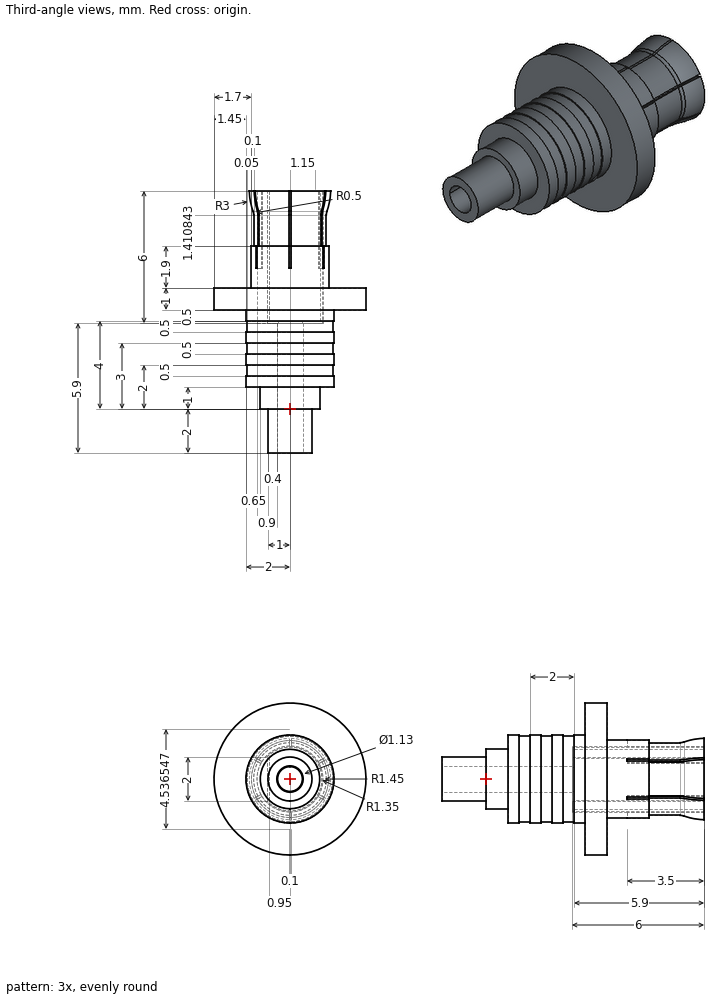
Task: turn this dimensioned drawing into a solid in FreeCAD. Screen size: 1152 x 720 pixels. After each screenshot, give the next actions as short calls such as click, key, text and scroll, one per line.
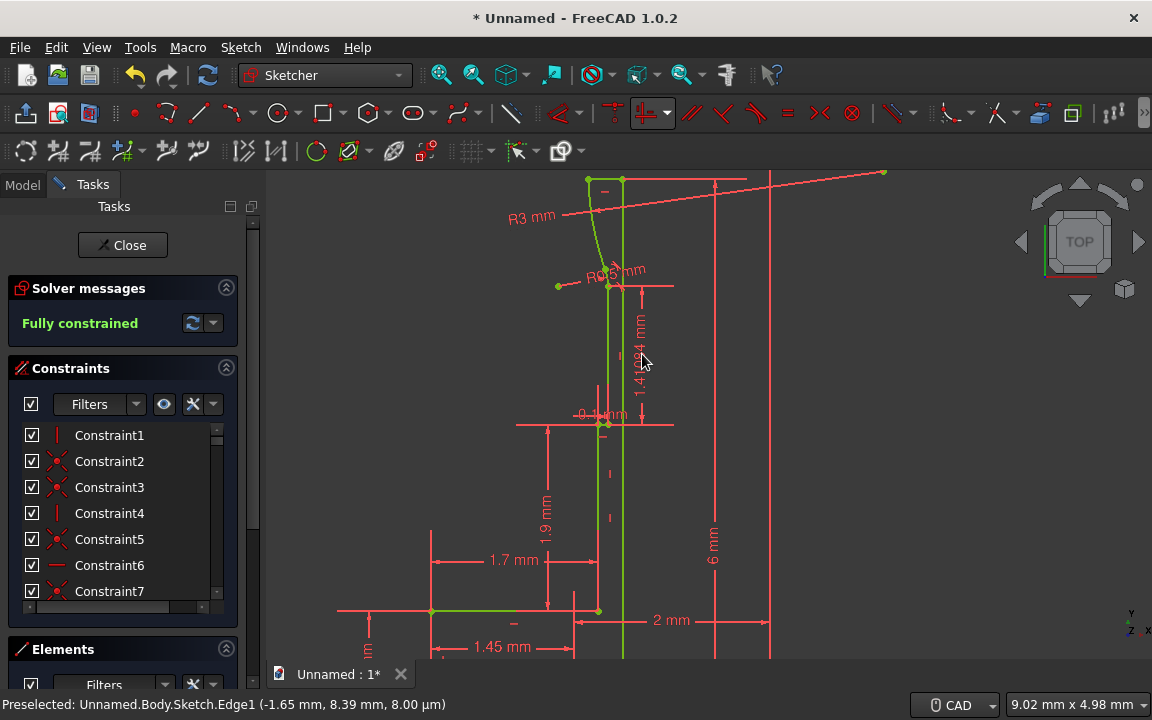
click(123, 245)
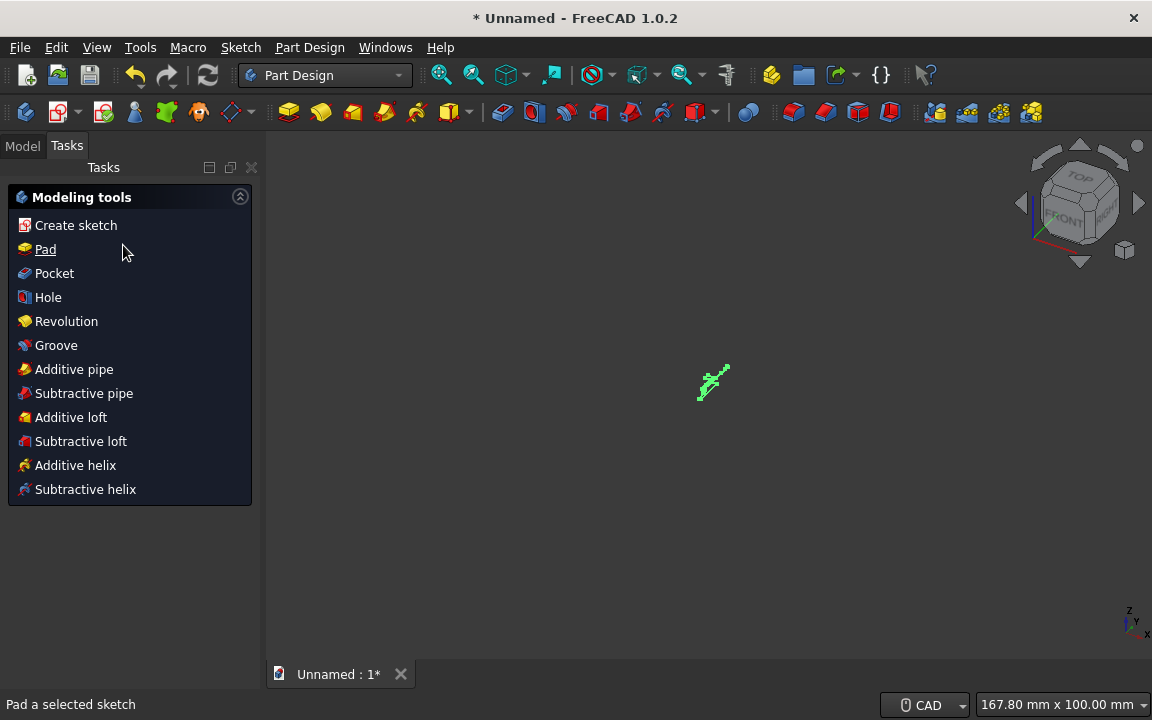
click(322, 112)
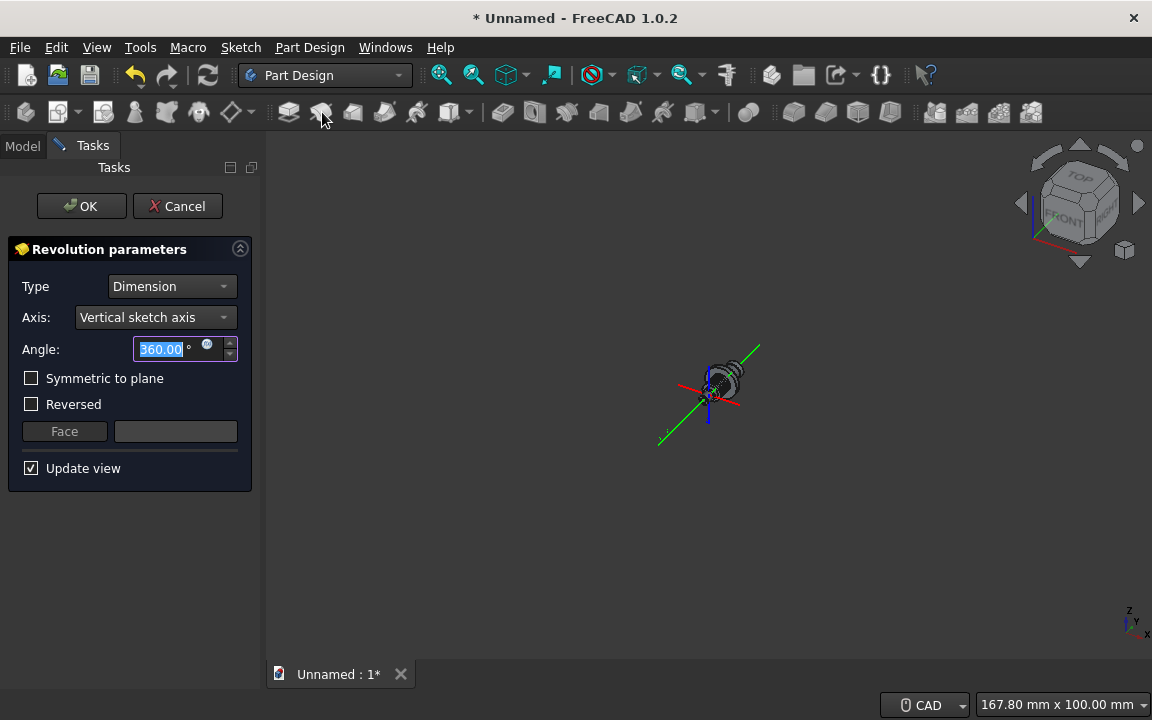
click(82, 206)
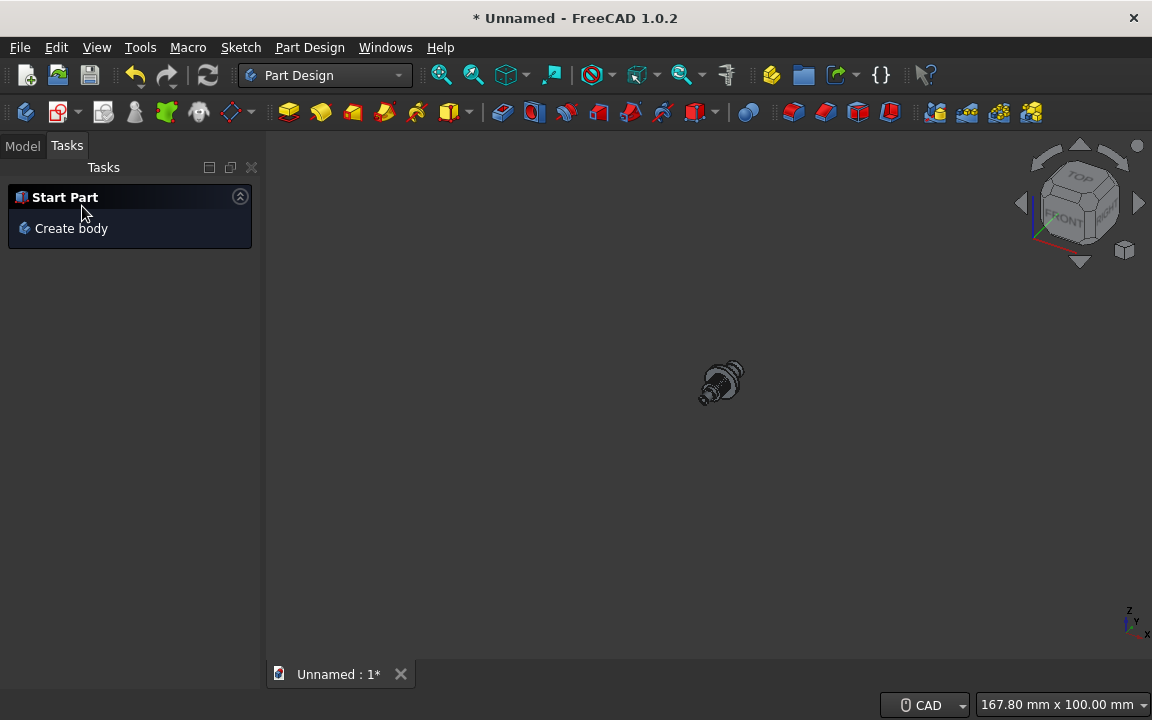
click(442, 76)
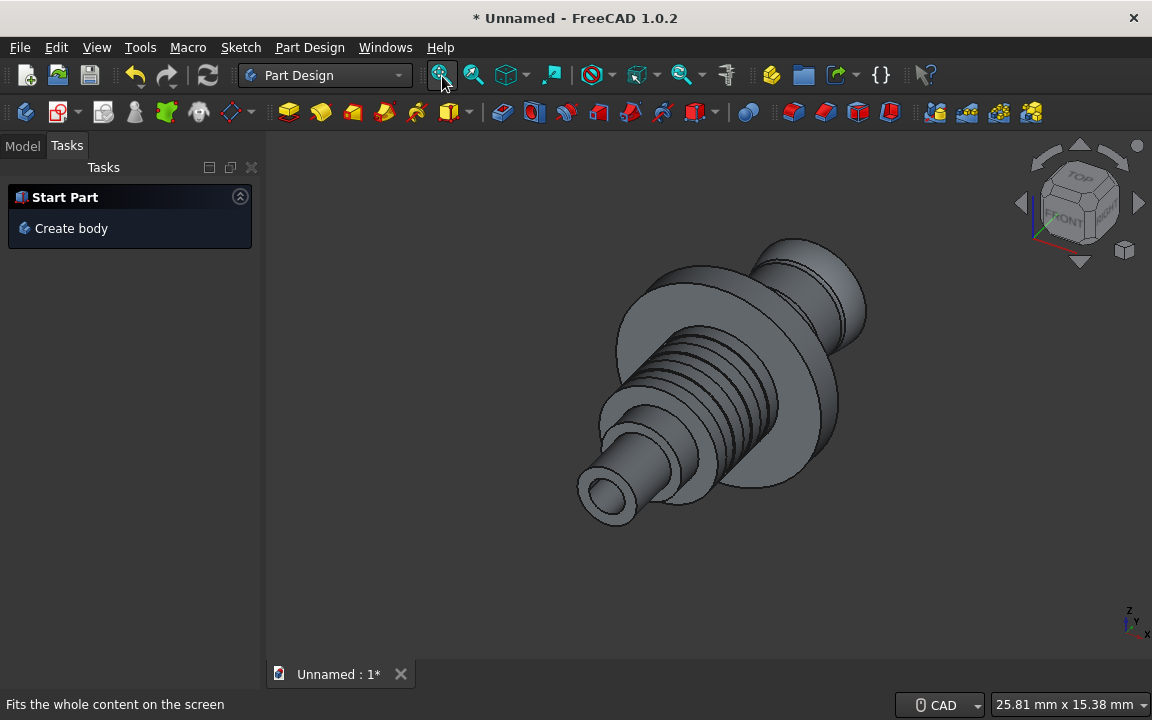
key(4)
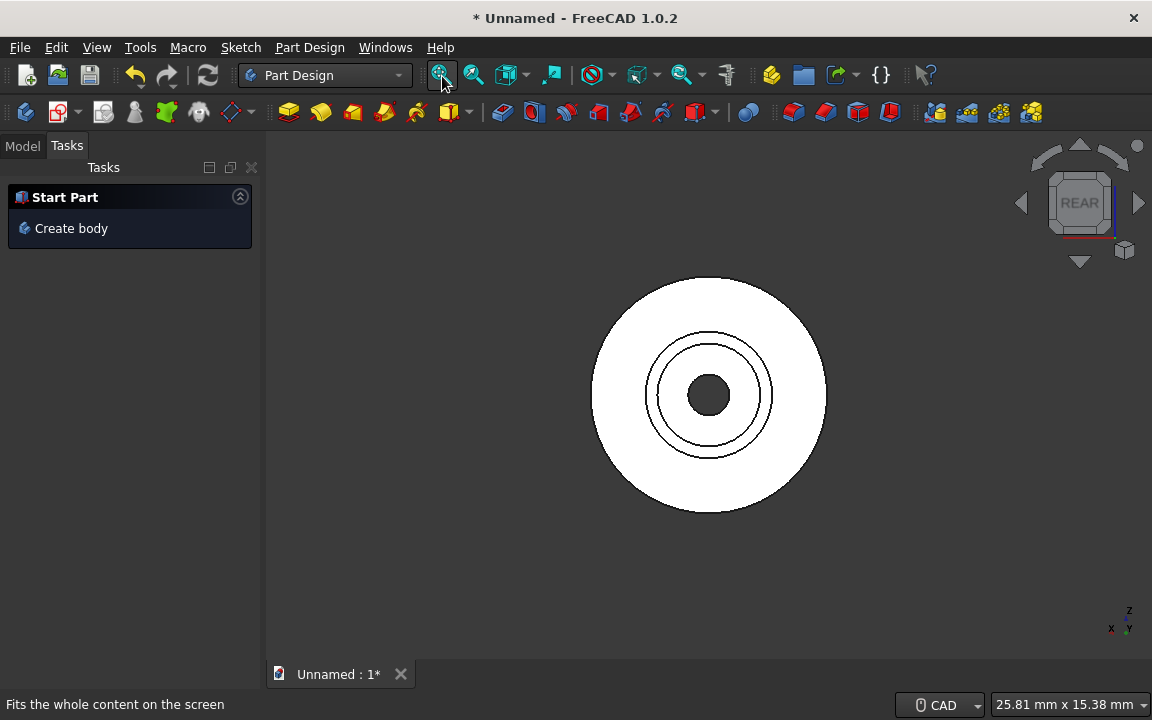
click(442, 76)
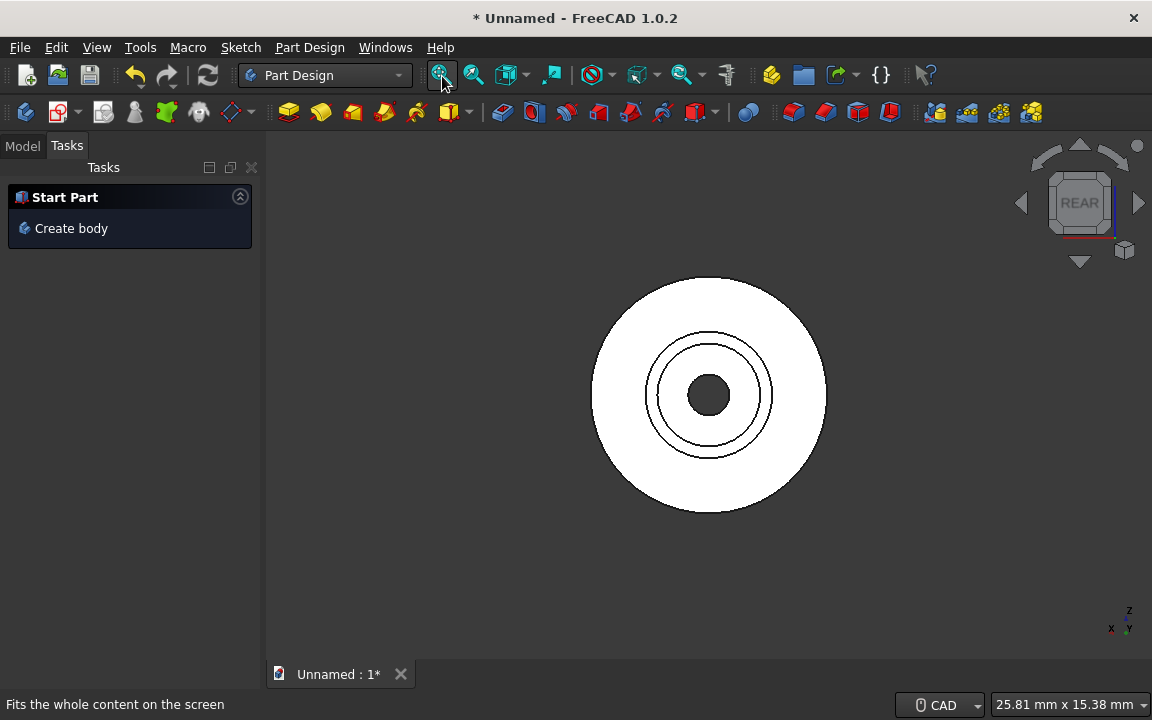
scroll(727, 340, up, 4)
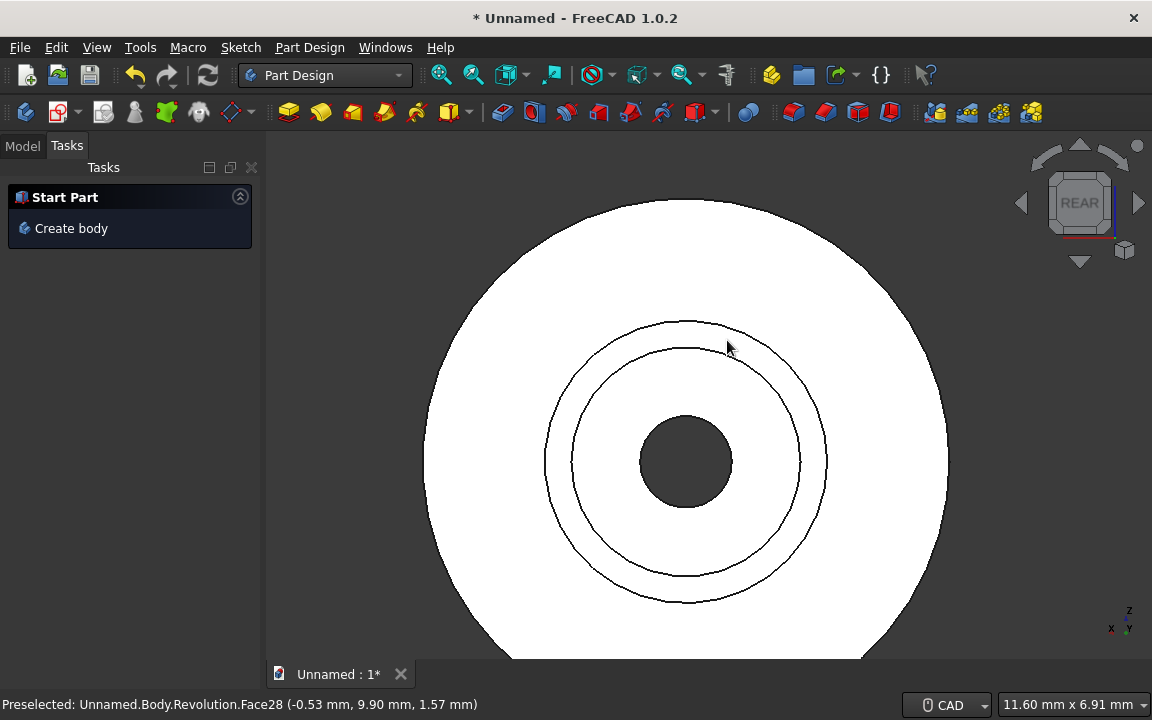
click(726, 340)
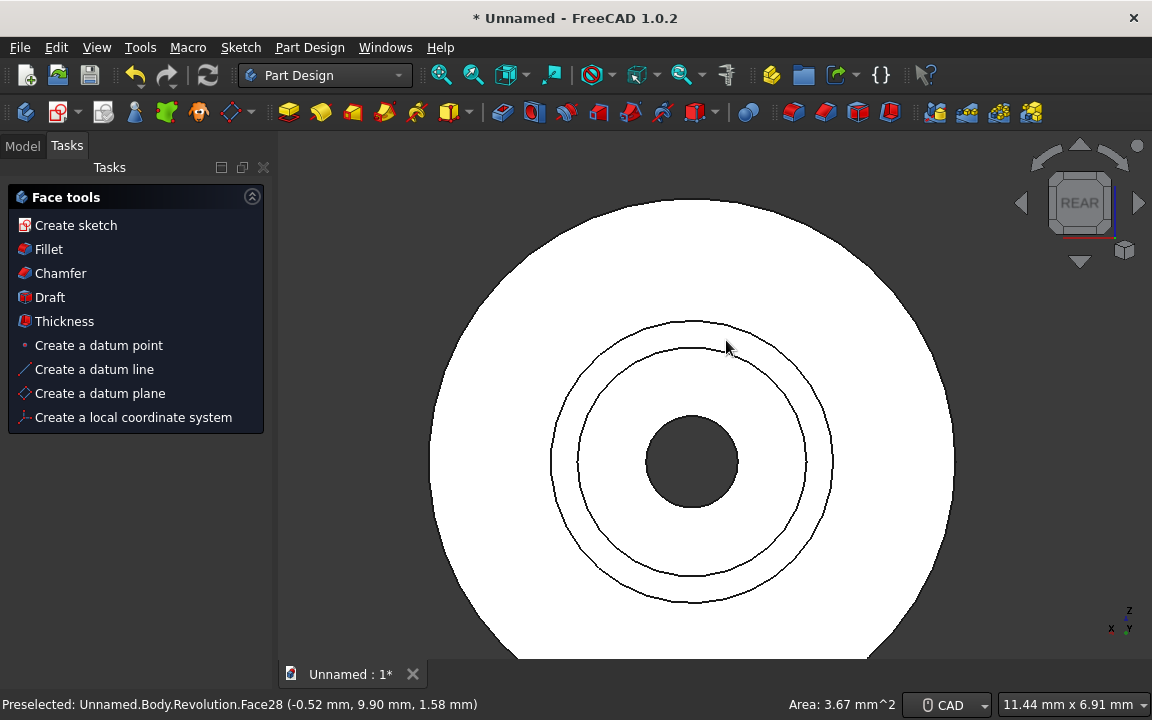
click(58, 112)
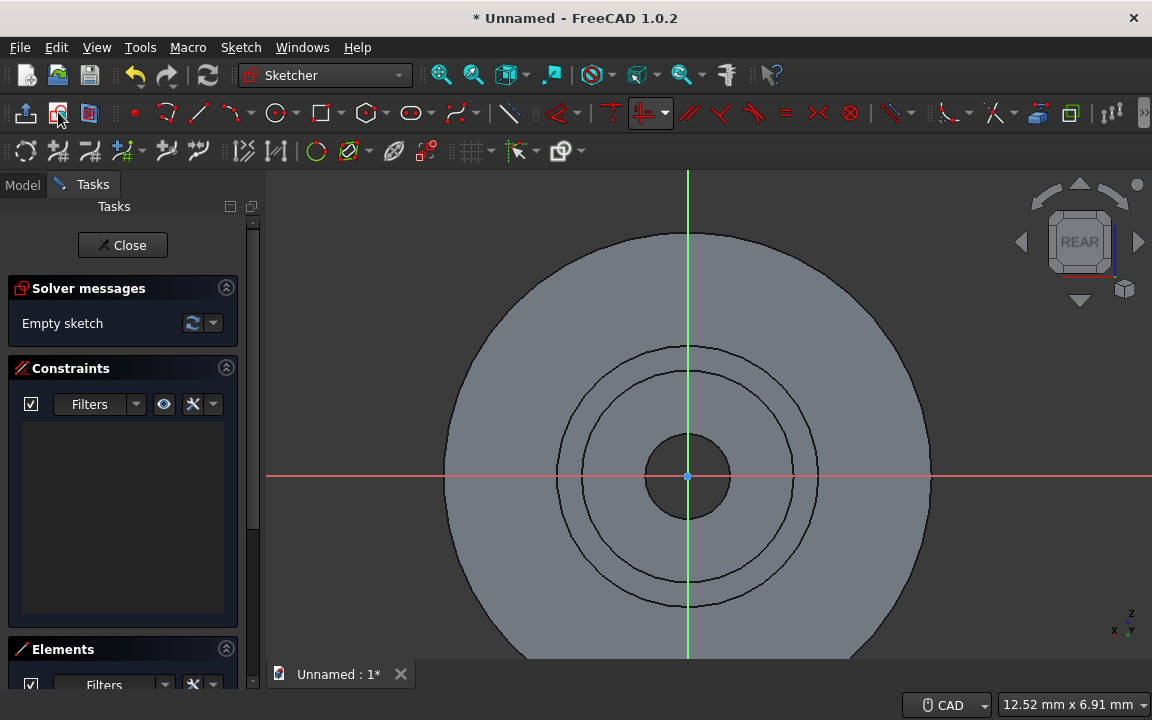
scroll(427, 198, down, 1)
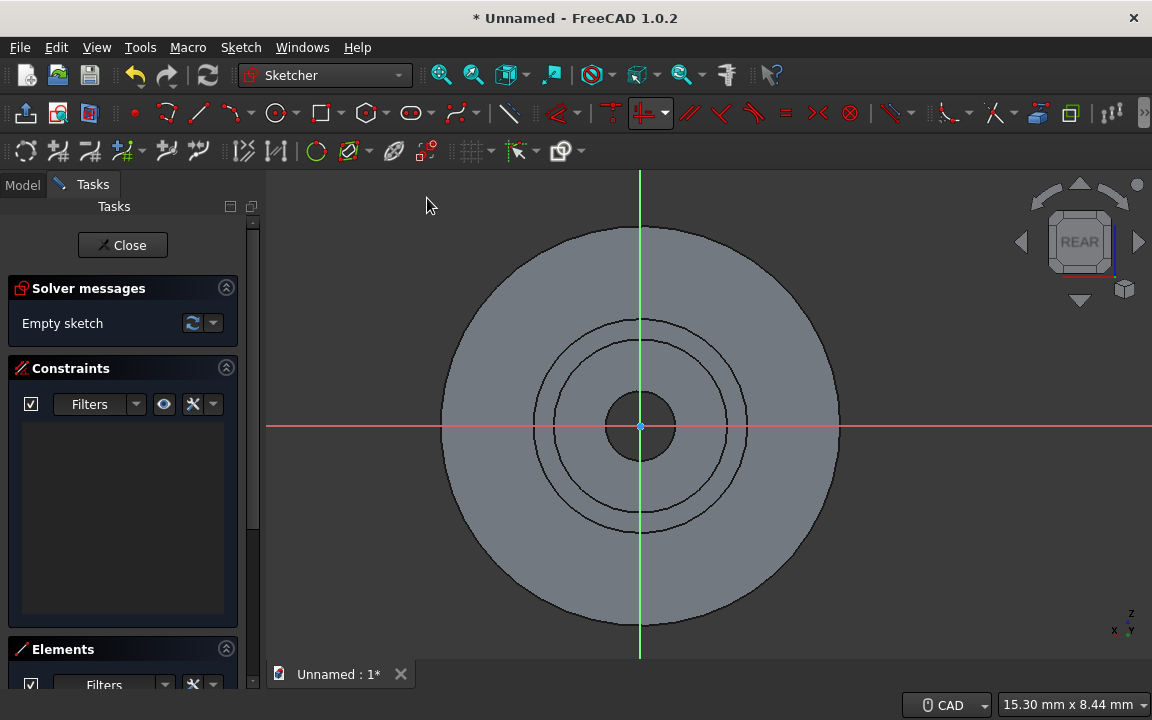
click(344, 114)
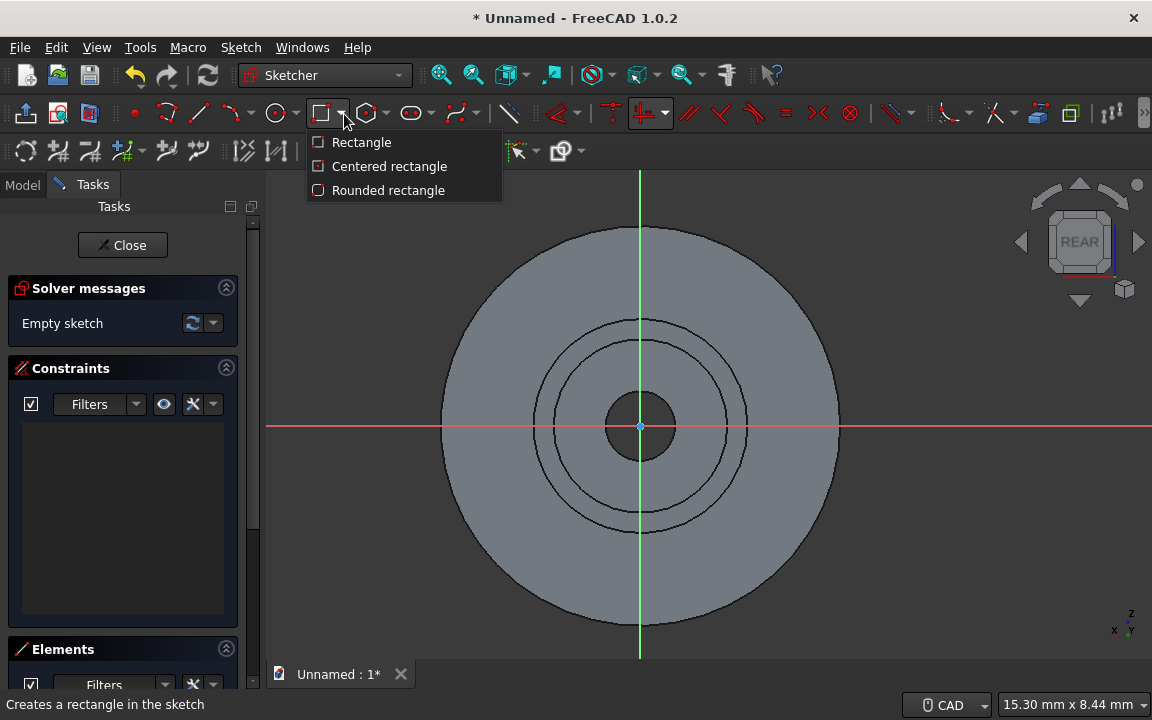
click(404, 166)